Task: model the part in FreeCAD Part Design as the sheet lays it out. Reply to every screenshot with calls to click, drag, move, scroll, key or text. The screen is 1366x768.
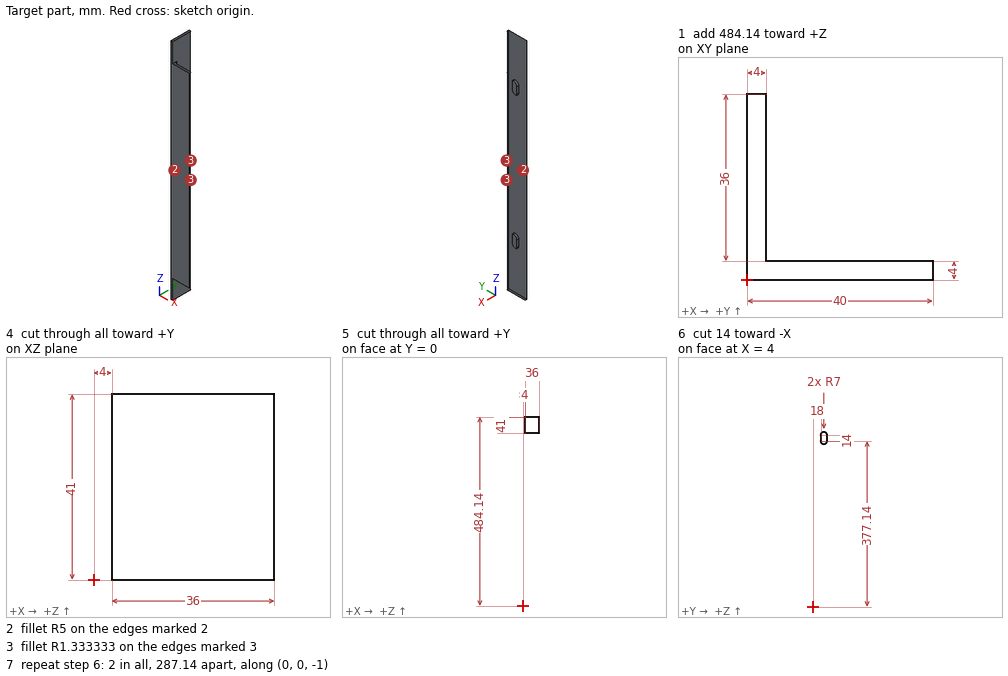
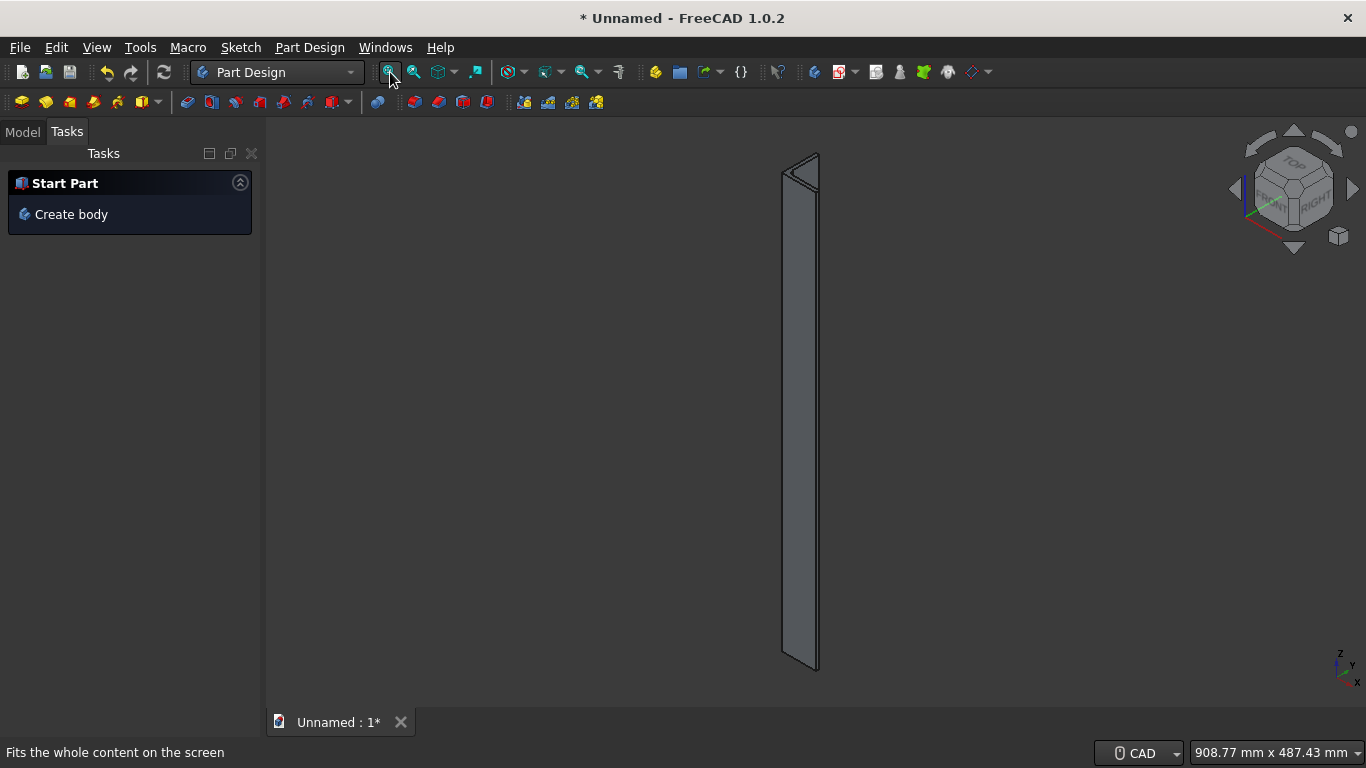
key(1)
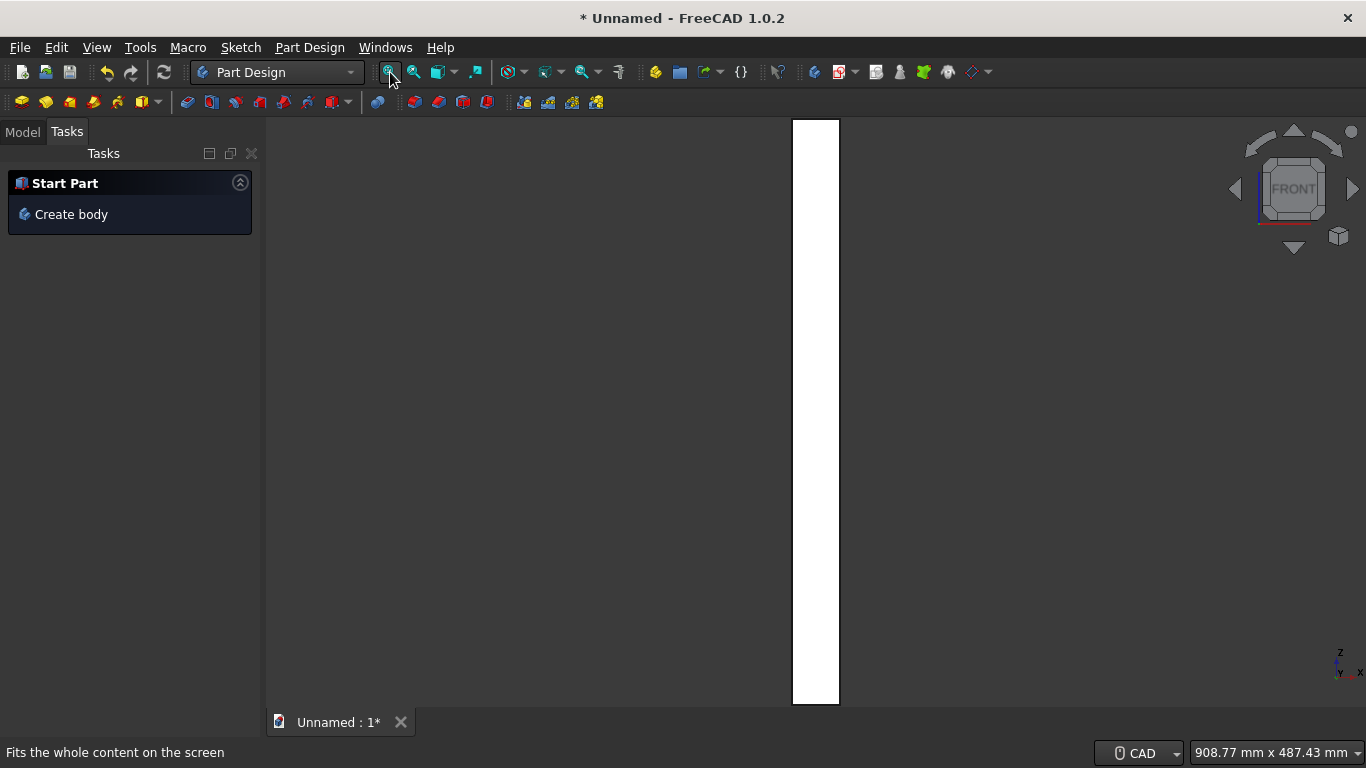
key(3)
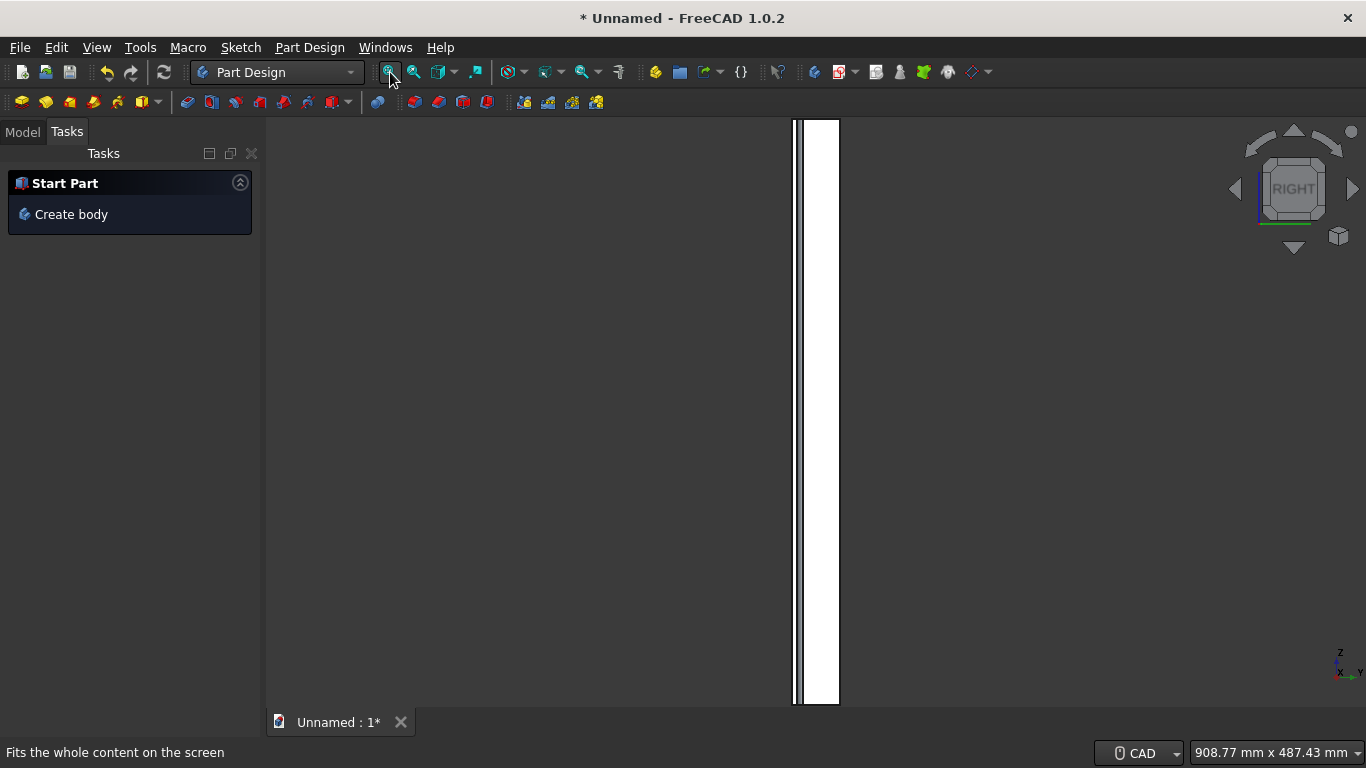
click(797, 411)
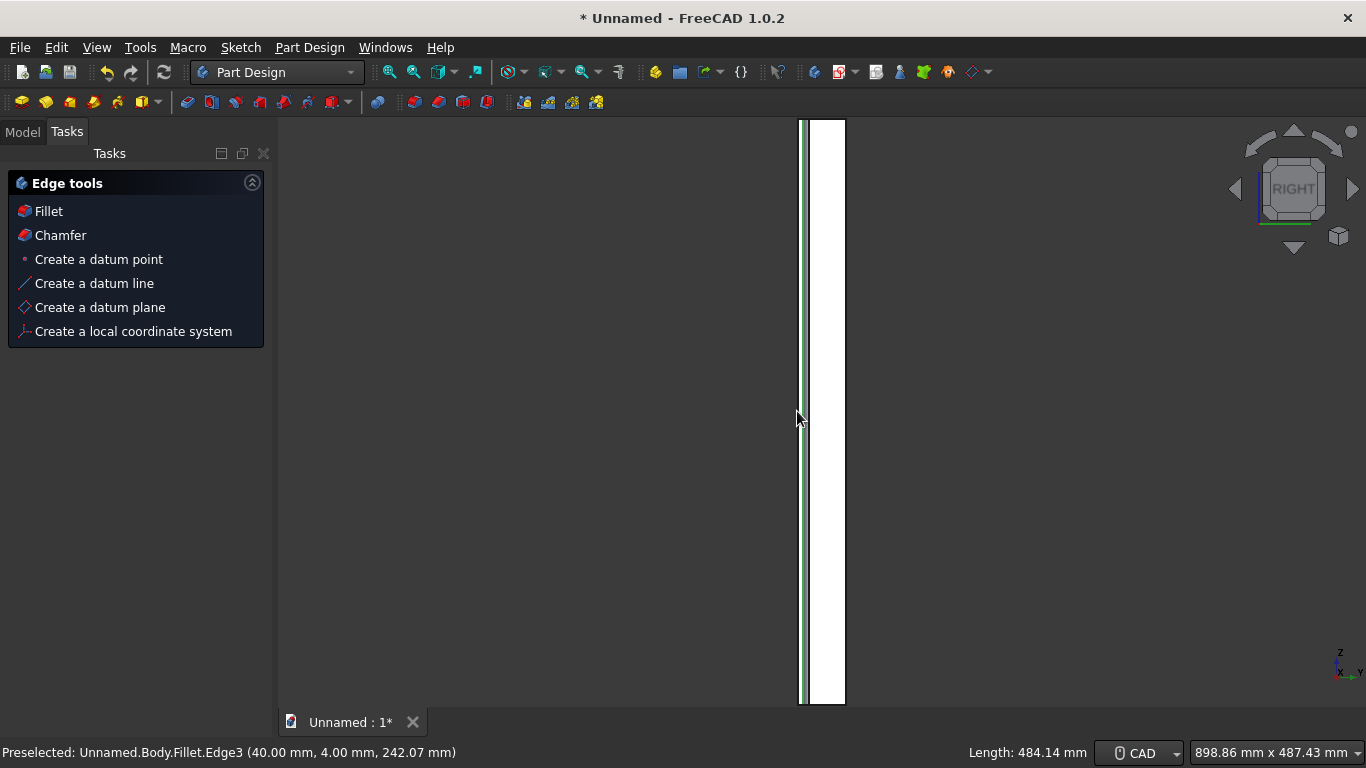
click(846, 411, ctrl)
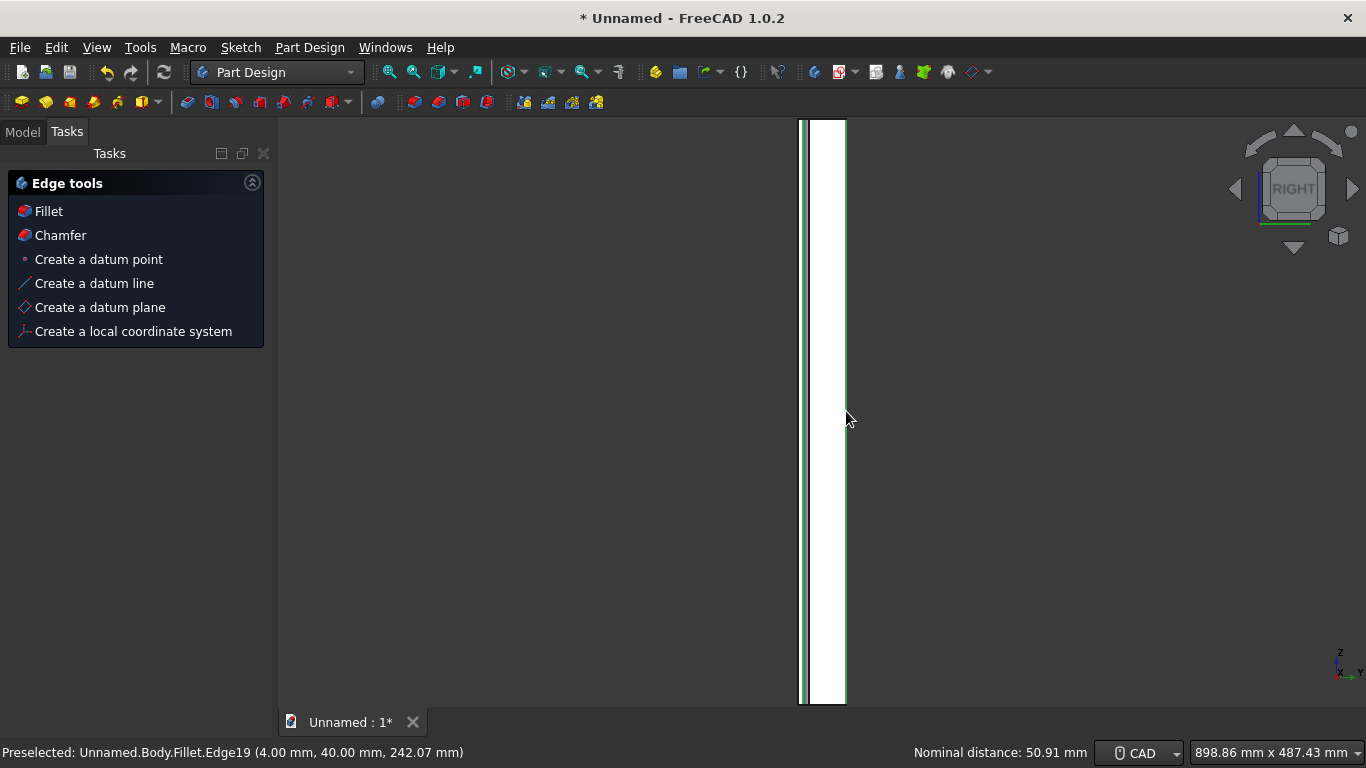
click(416, 102)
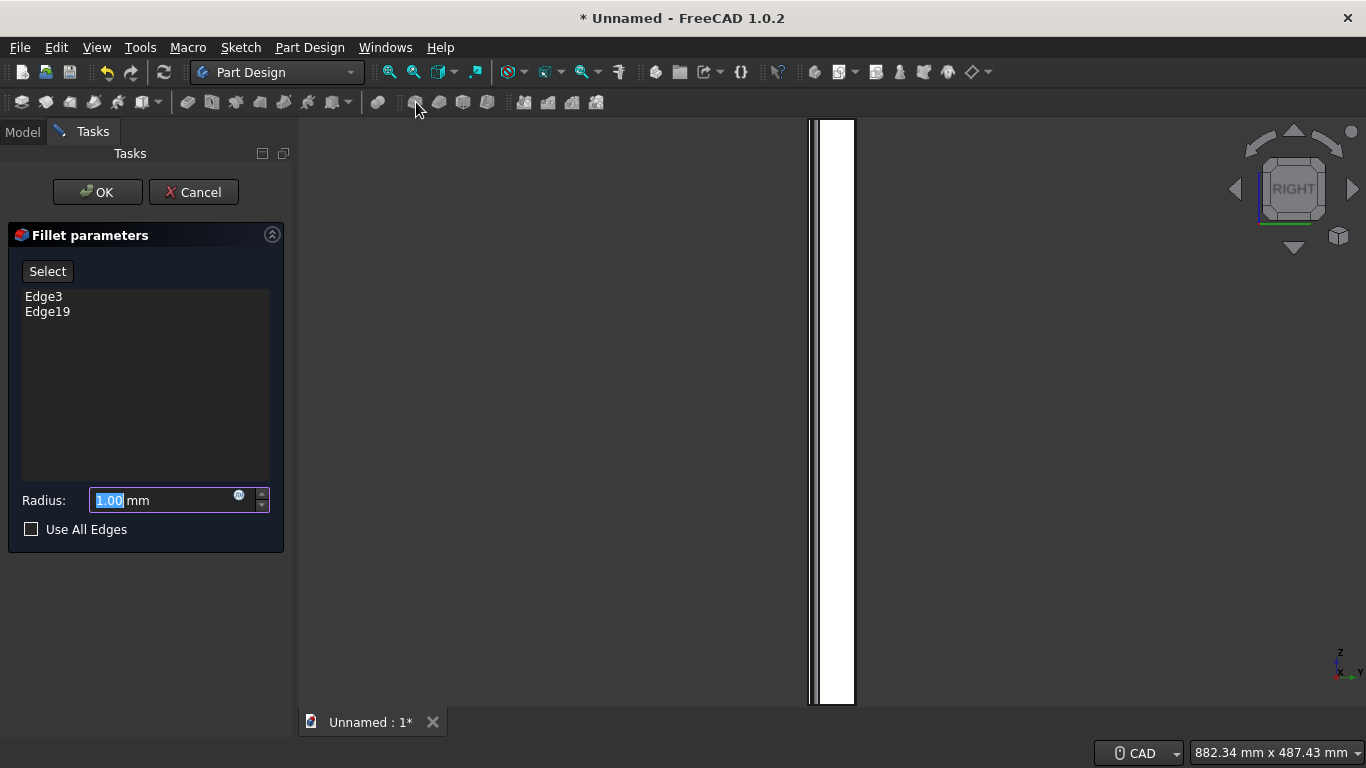
text(1.333333)
key(Tab)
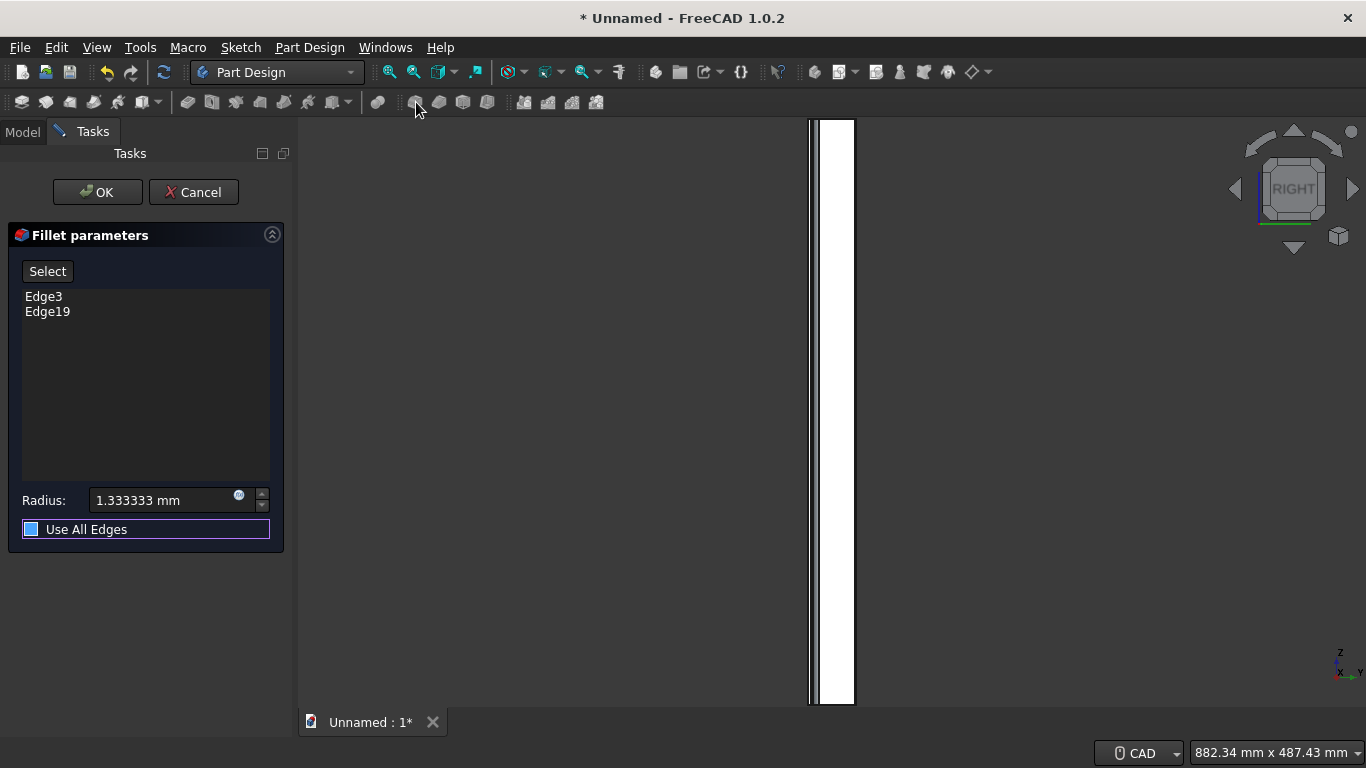
click(98, 192)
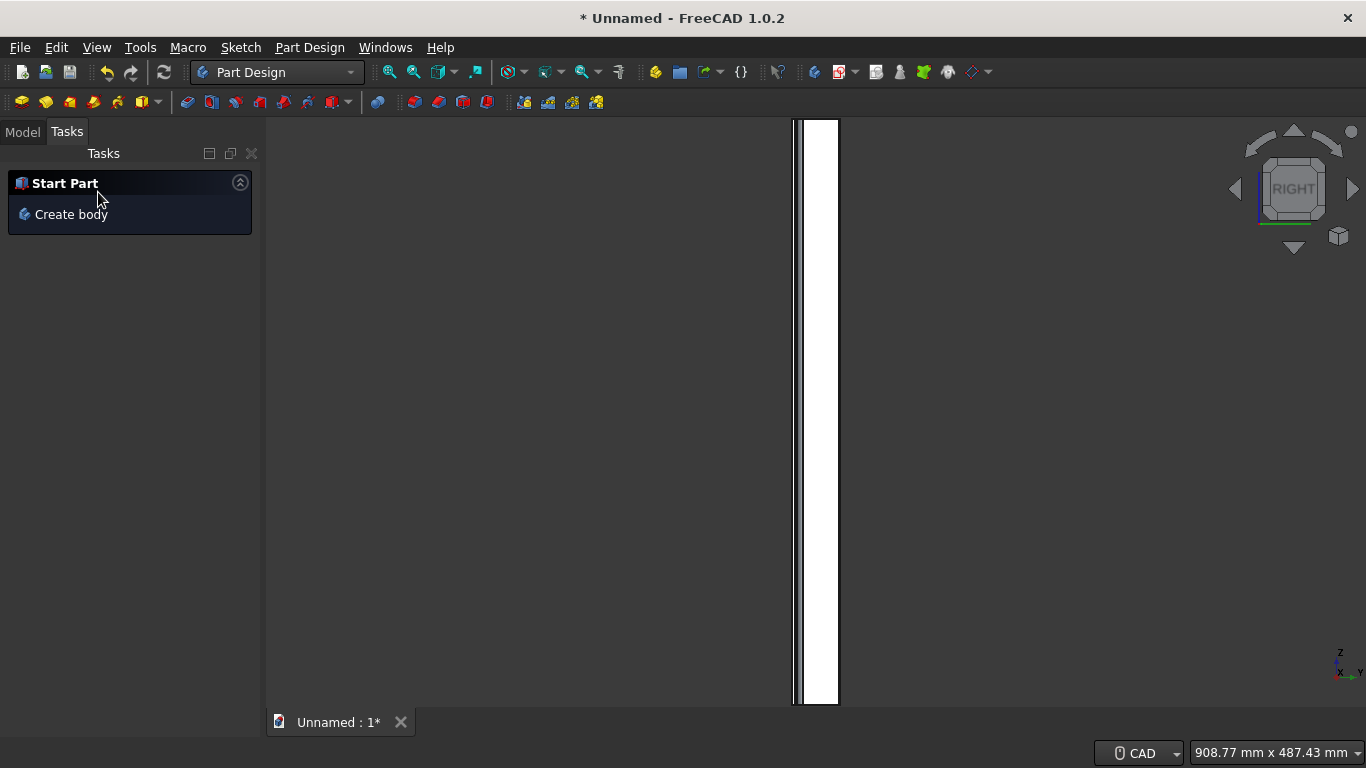
click(840, 72)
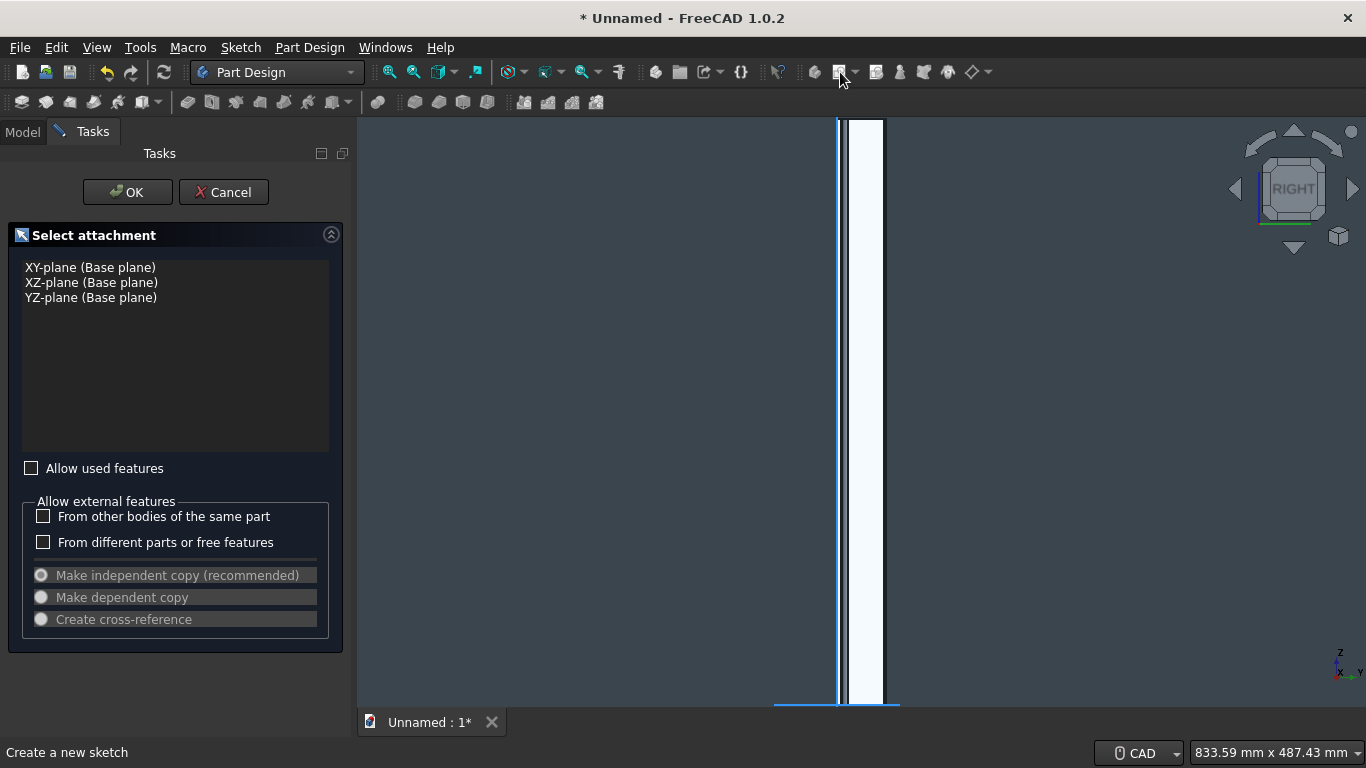
click(82, 282)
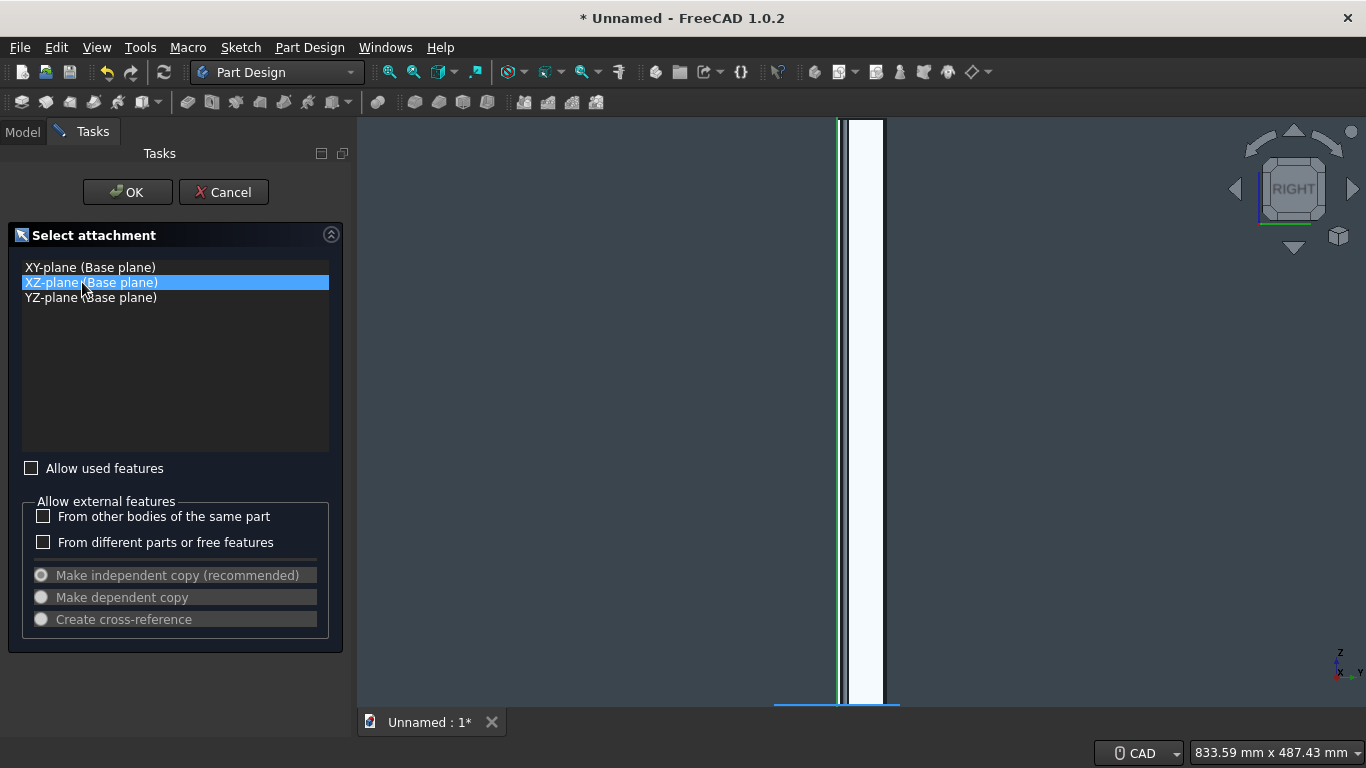
click(128, 192)